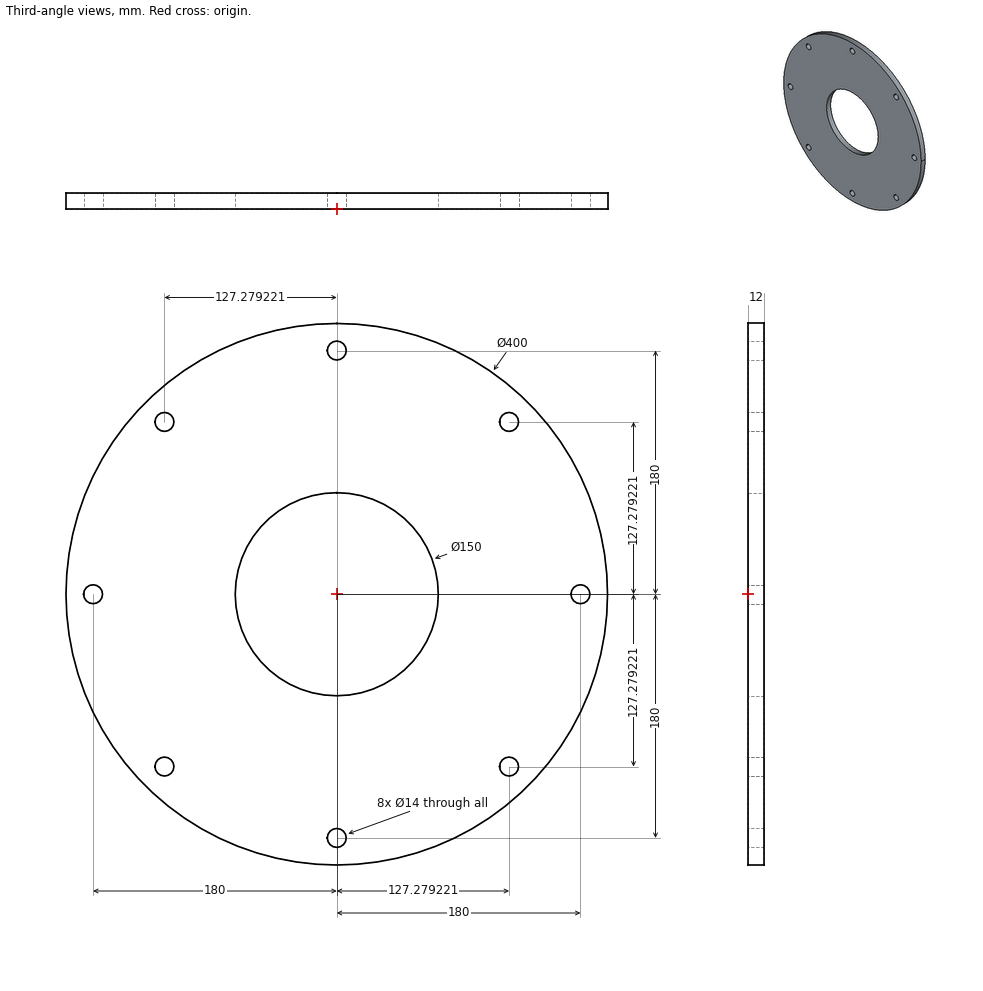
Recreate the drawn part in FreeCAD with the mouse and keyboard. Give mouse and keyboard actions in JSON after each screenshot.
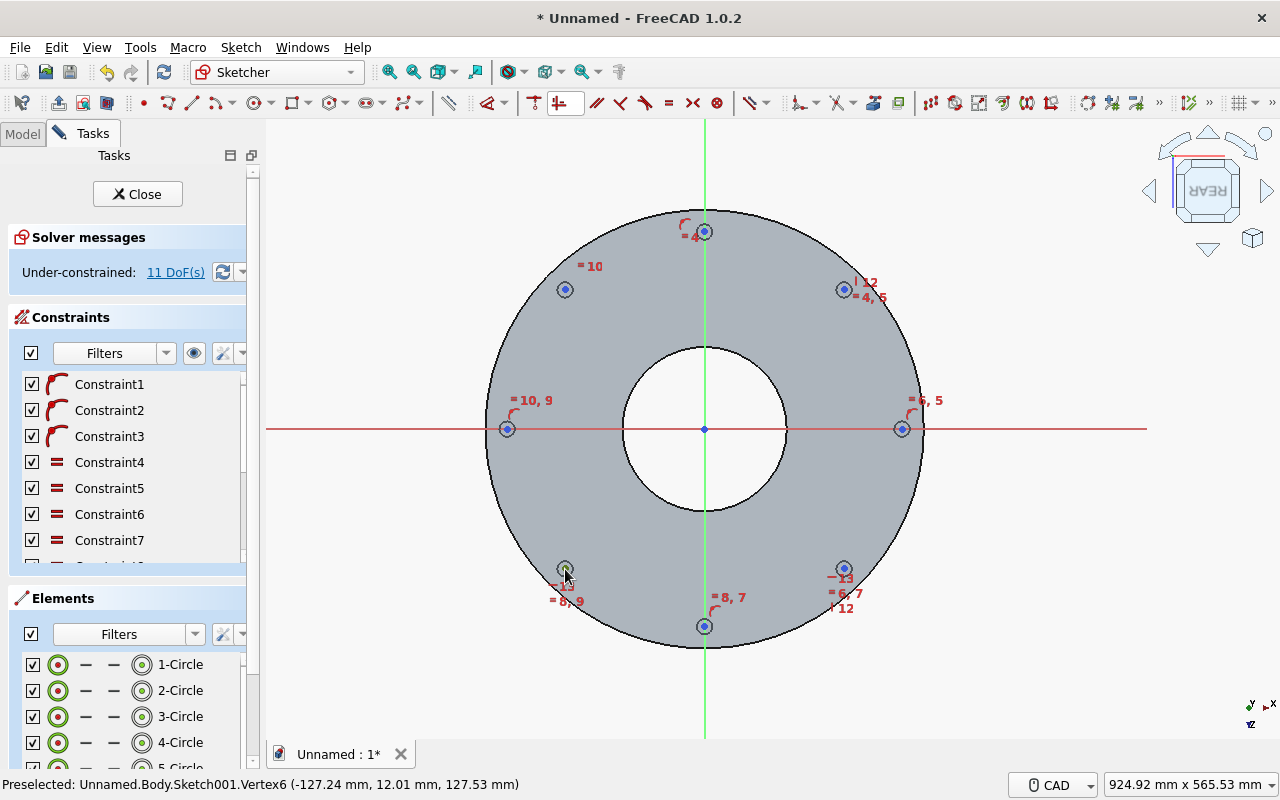
{"action": "left_click", "coordinate": [565, 290]}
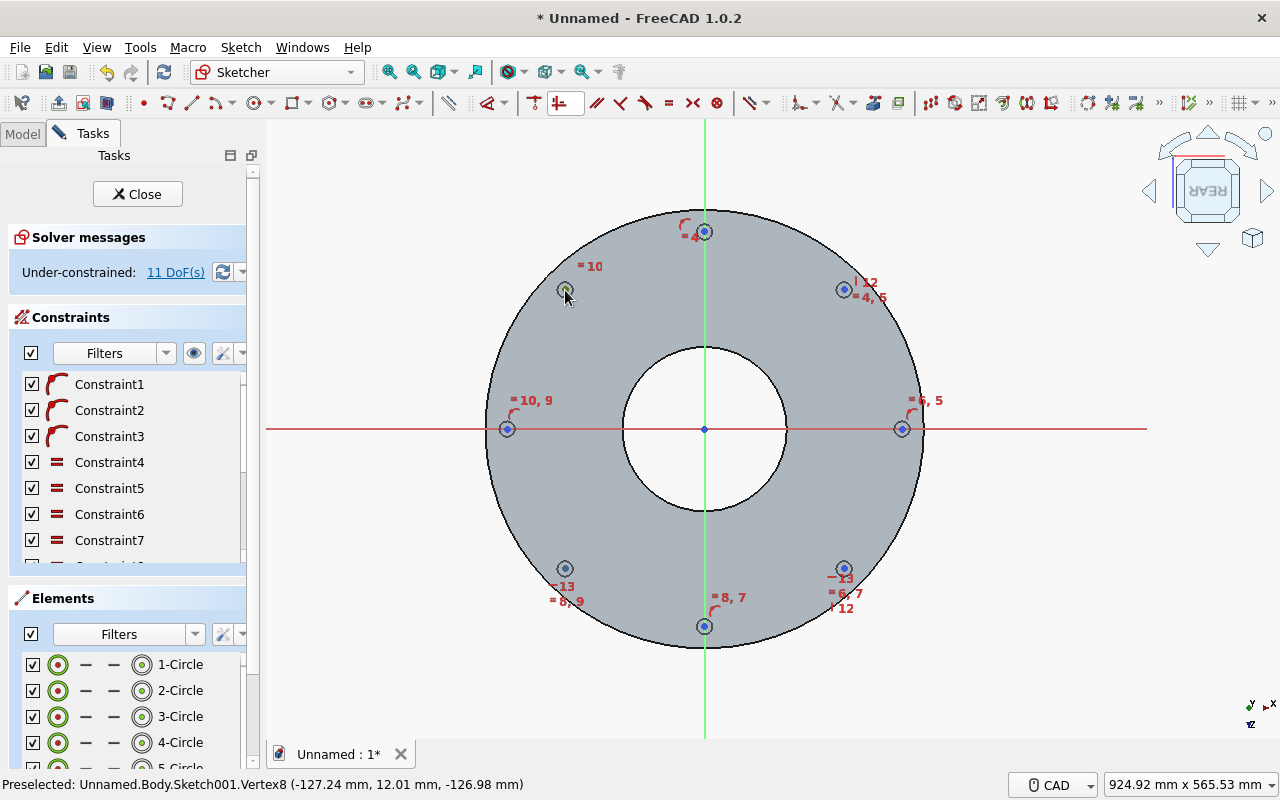
{"action": "key", "text": "v"}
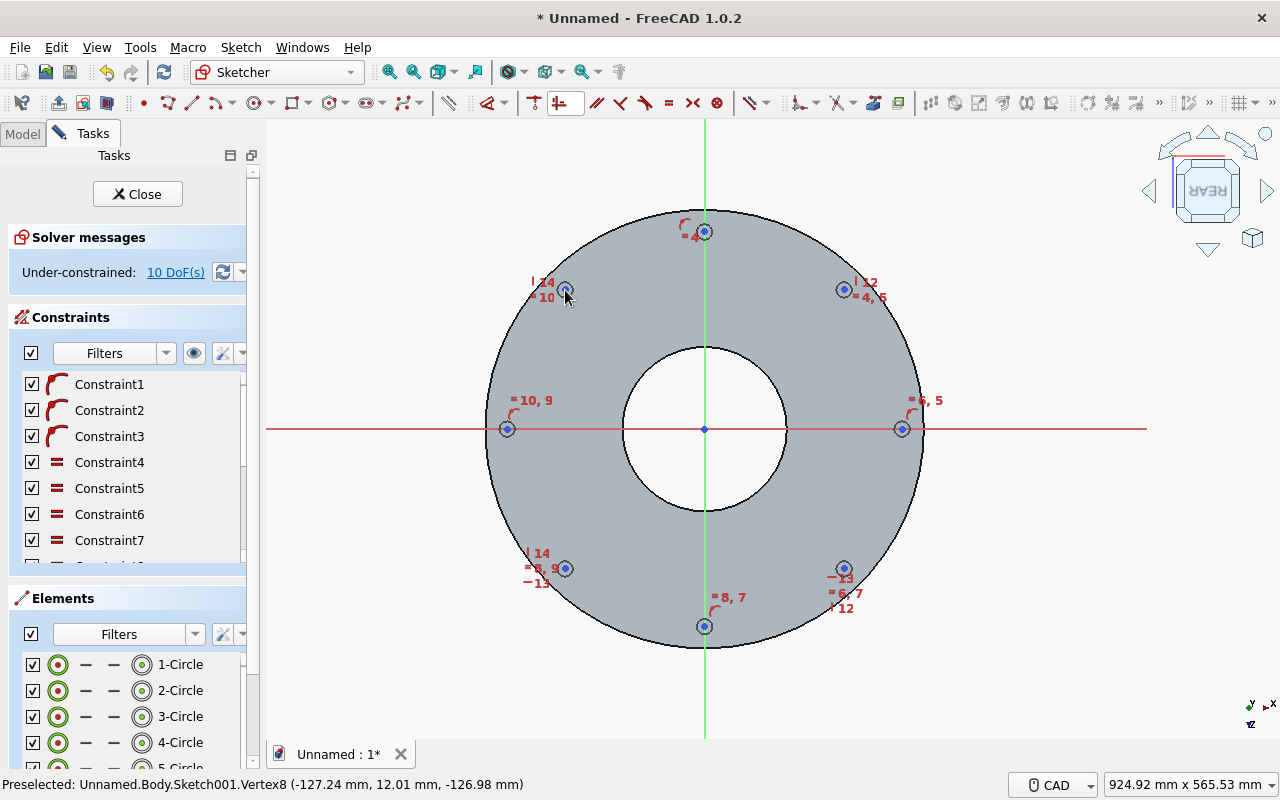
{"action": "left_click", "coordinate": [844, 290]}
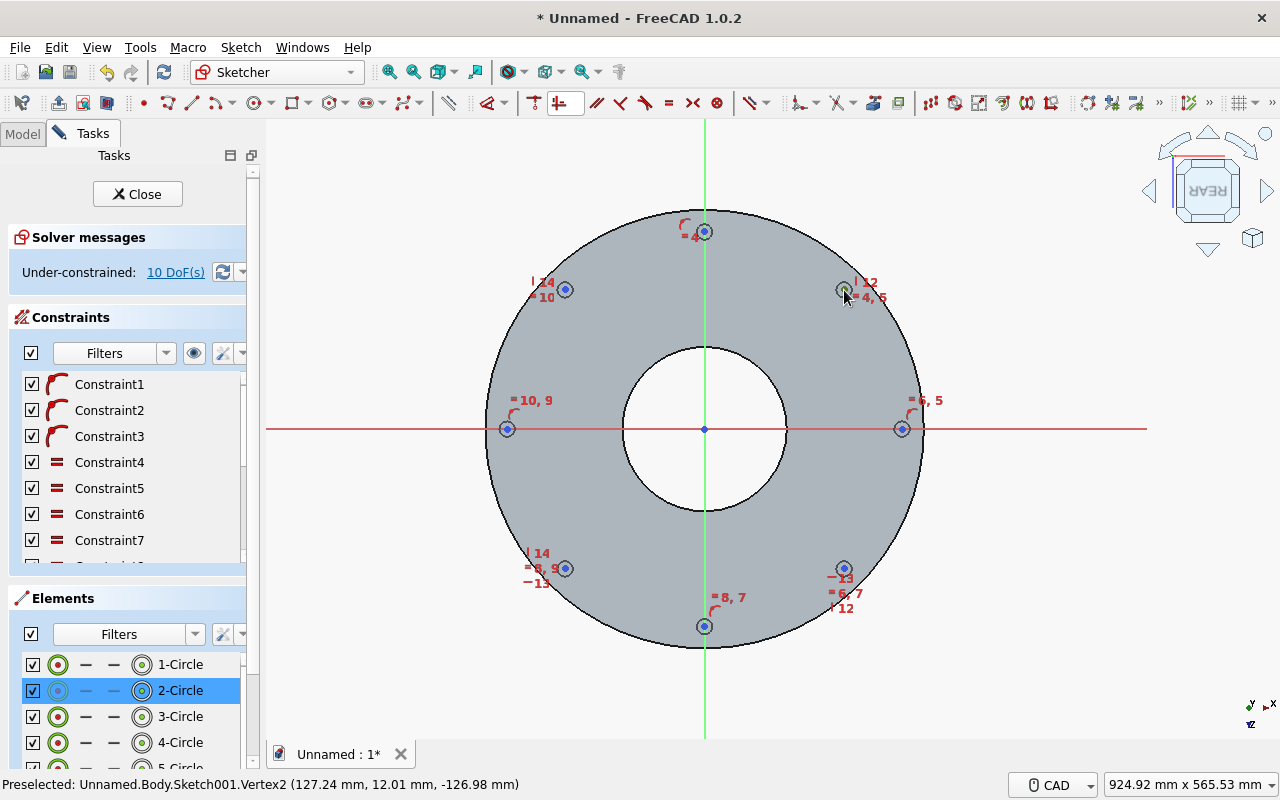
{"action": "left_click", "coordinate": [565, 290]}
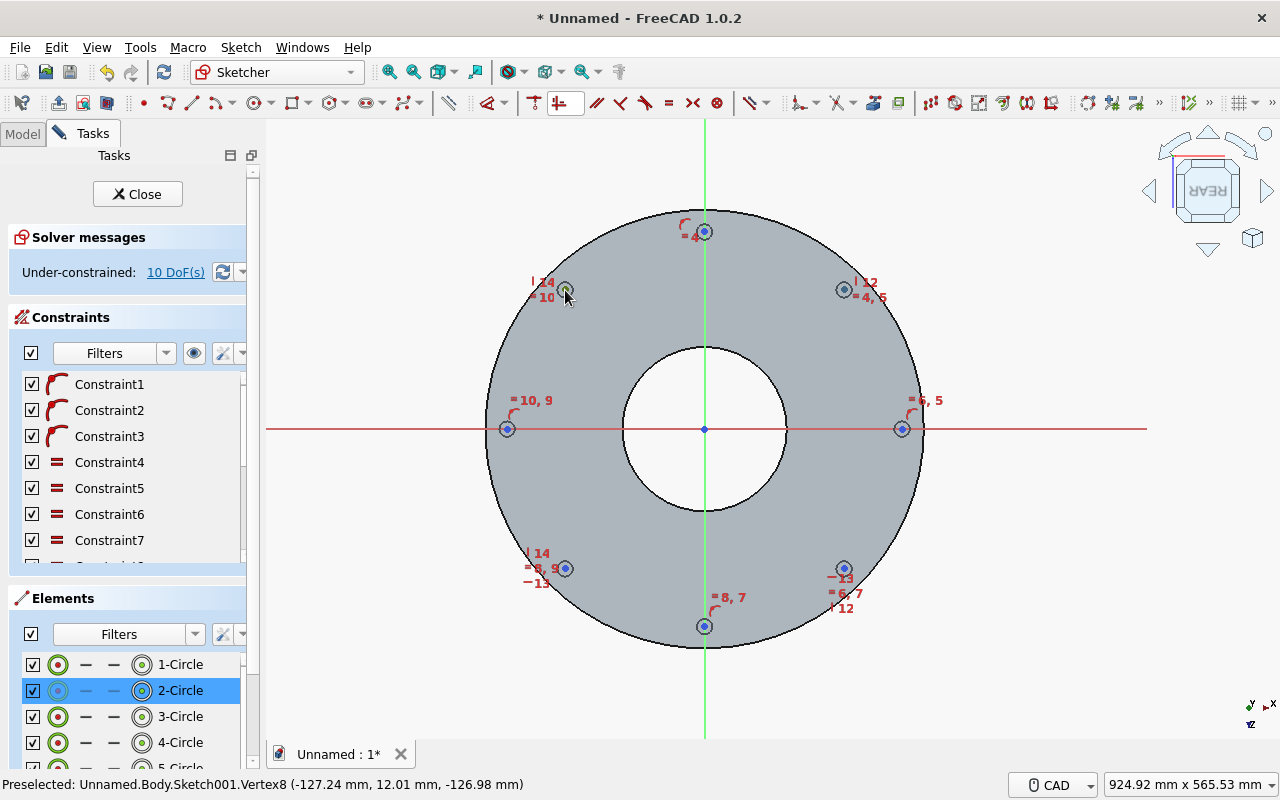
{"action": "left_click", "coordinate": [578, 104]}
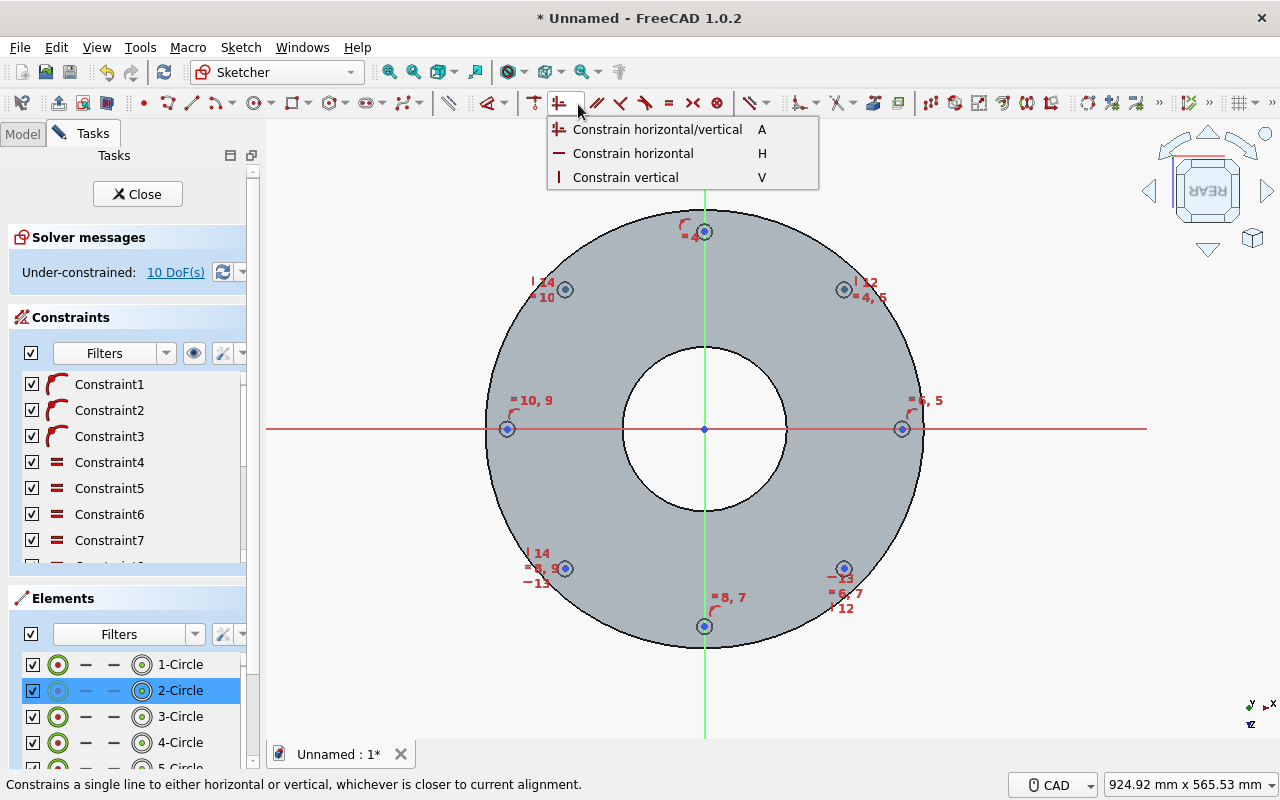
{"action": "left_click", "coordinate": [683, 153]}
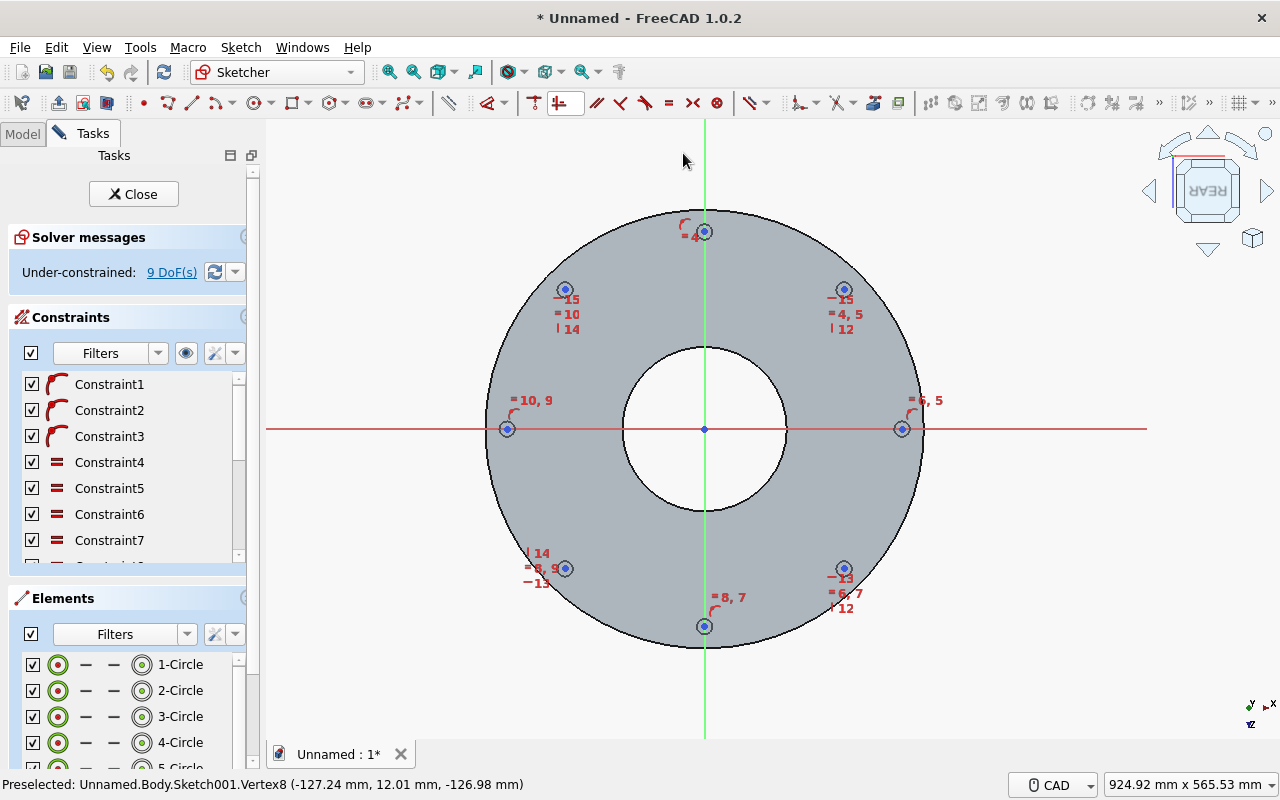
{"action": "left_click", "coordinate": [488, 104]}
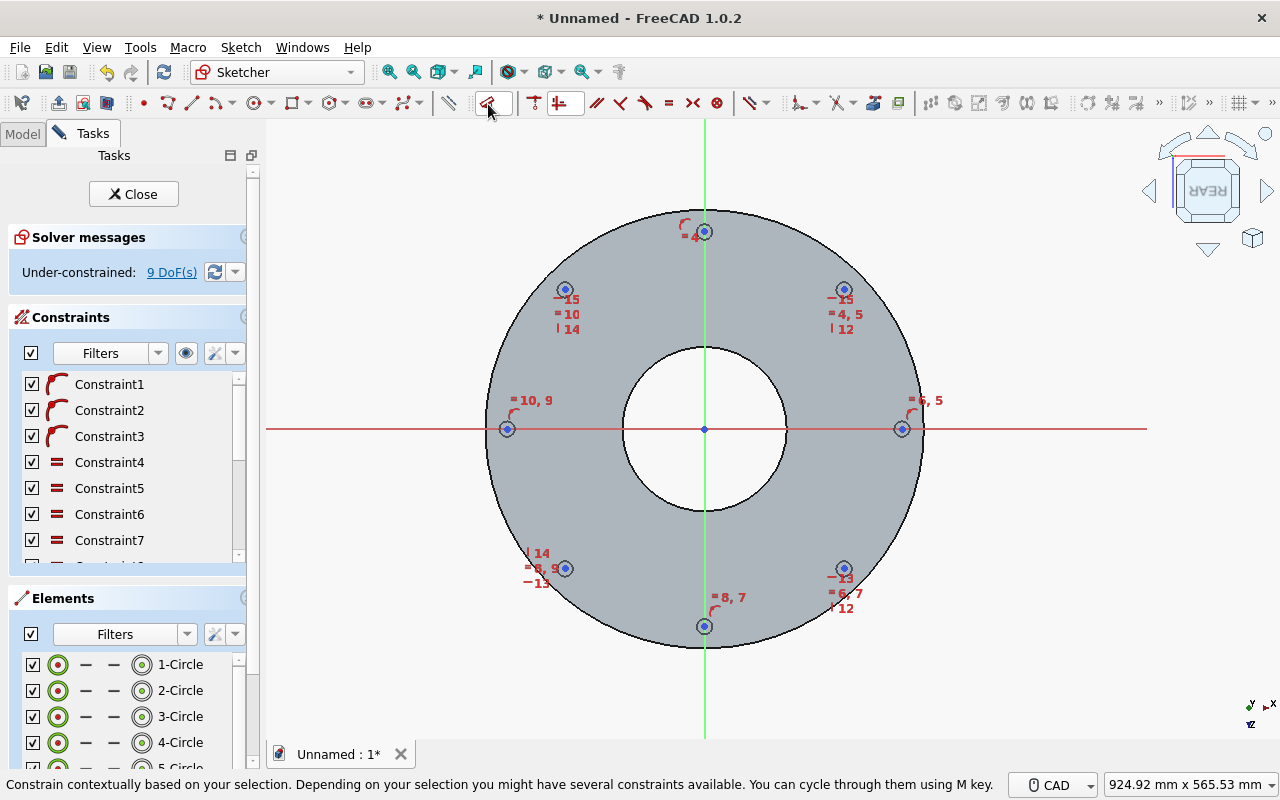
{"action": "scroll", "coordinate": [705, 224], "scroll_direction": "up", "scroll_amount": 5}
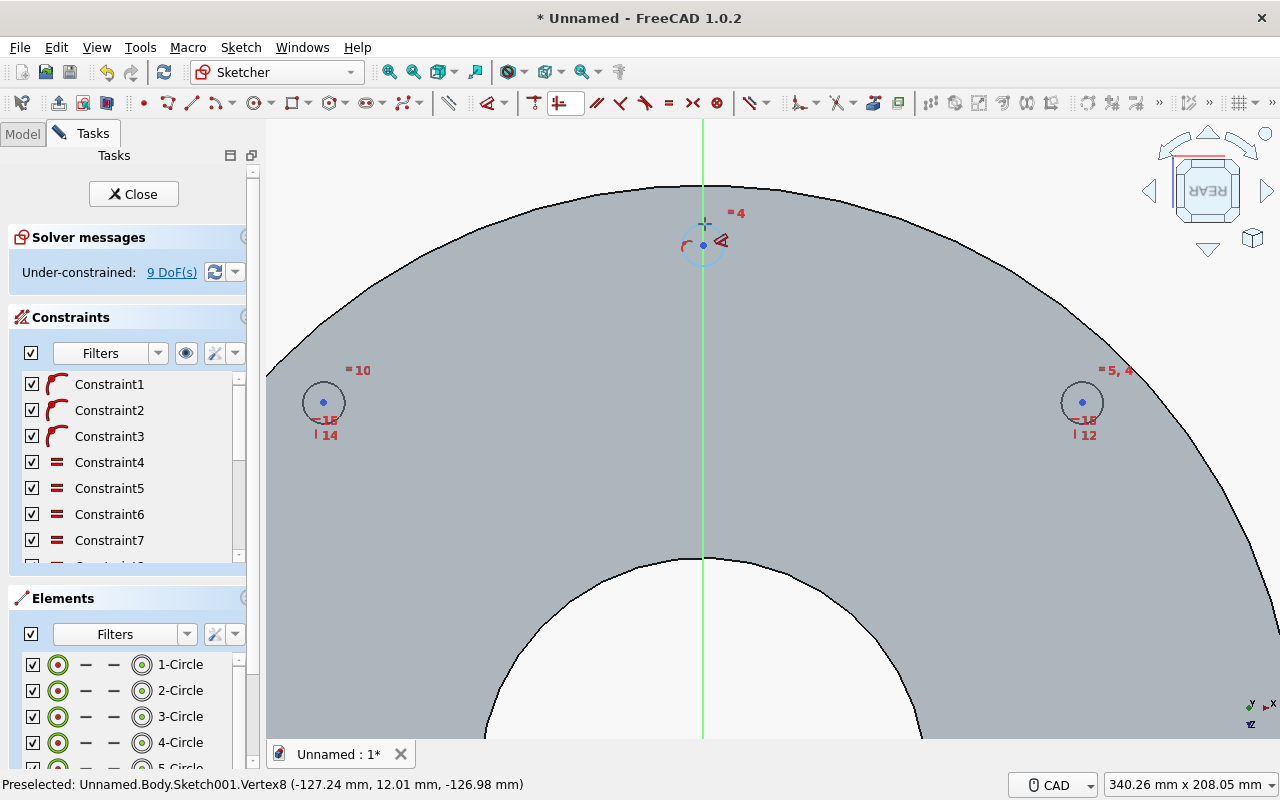
{"action": "left_click", "coordinate": [704, 225]}
{"action": "left_click", "coordinate": [730, 201]}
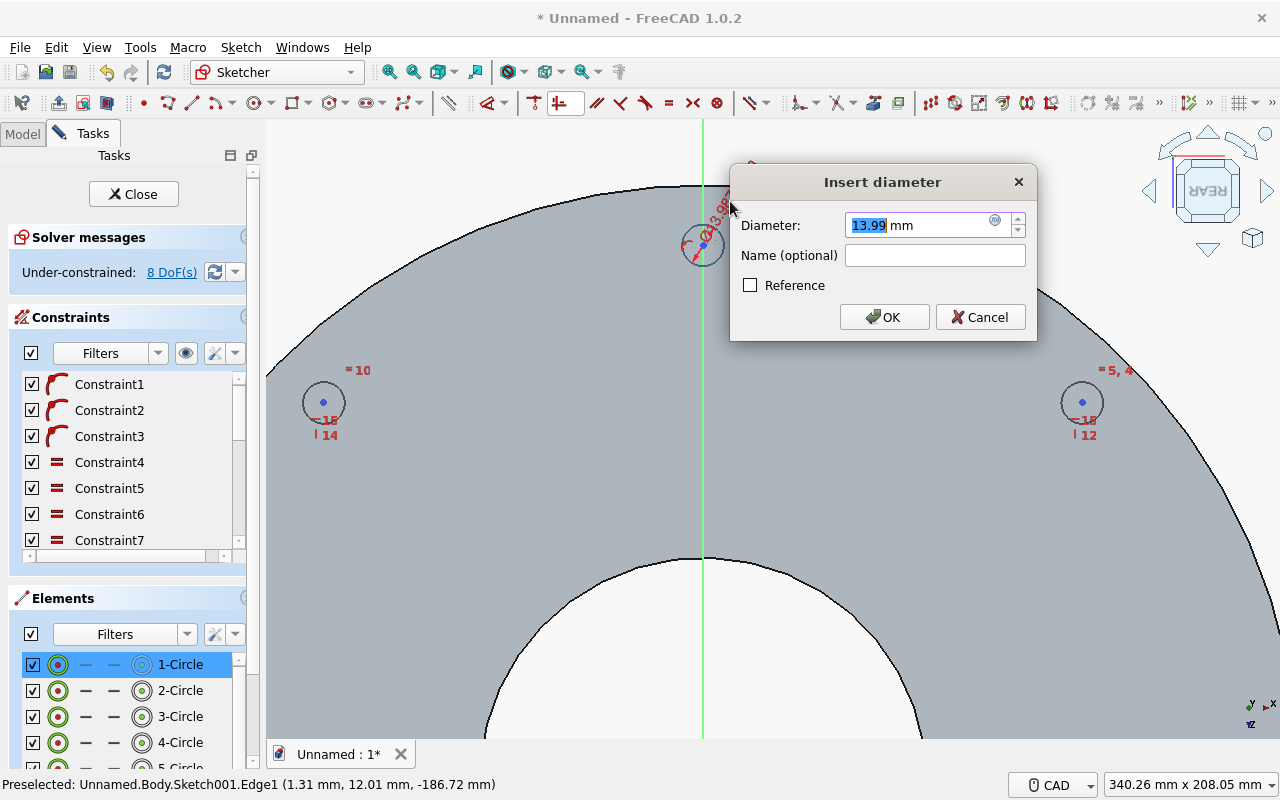
{"action": "type", "text": "14"}
{"action": "key", "text": "Return"}